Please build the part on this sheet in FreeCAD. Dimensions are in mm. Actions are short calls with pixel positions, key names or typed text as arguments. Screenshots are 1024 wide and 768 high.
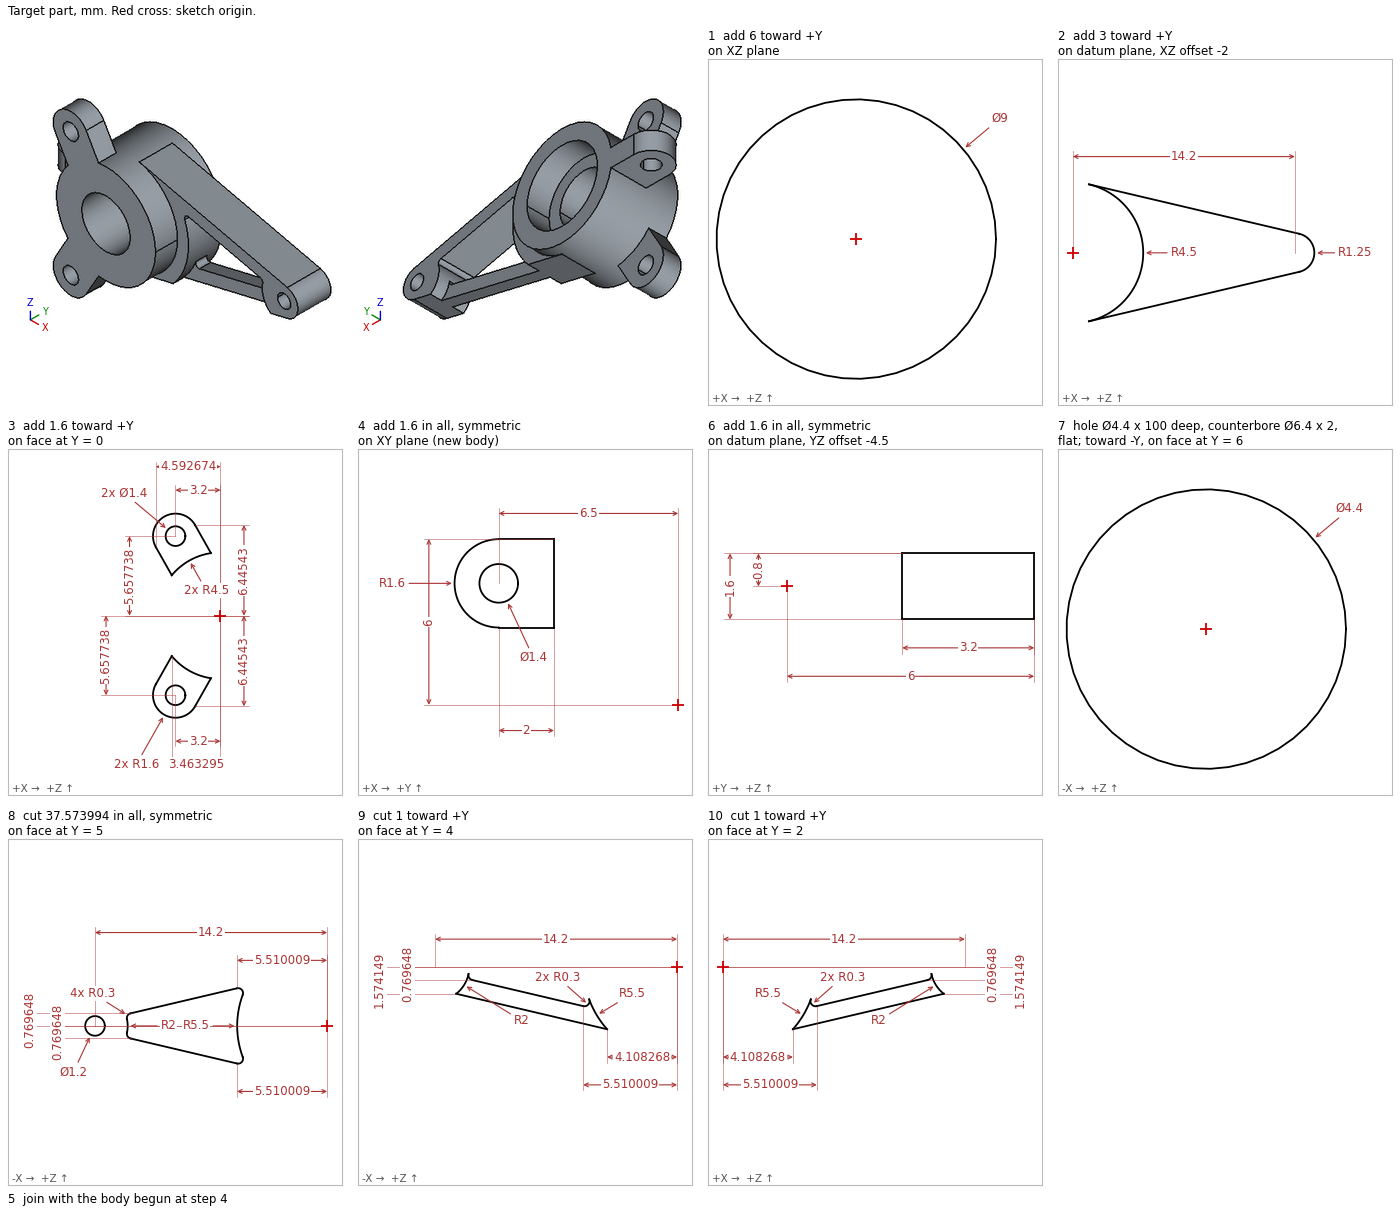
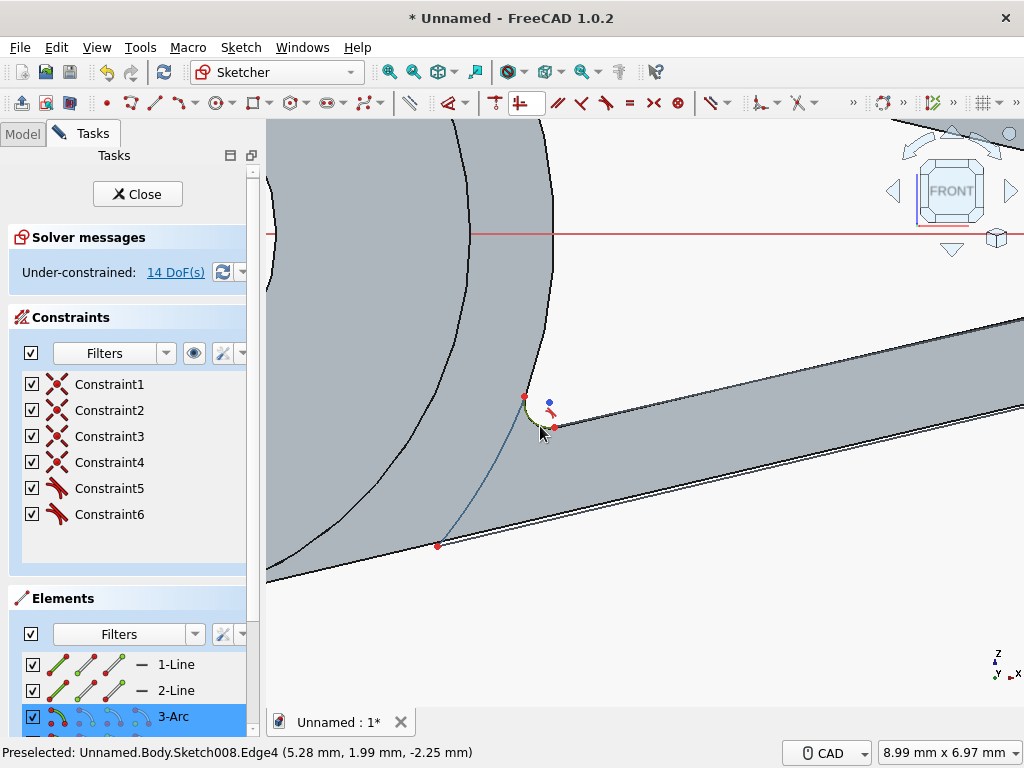
click(606, 104)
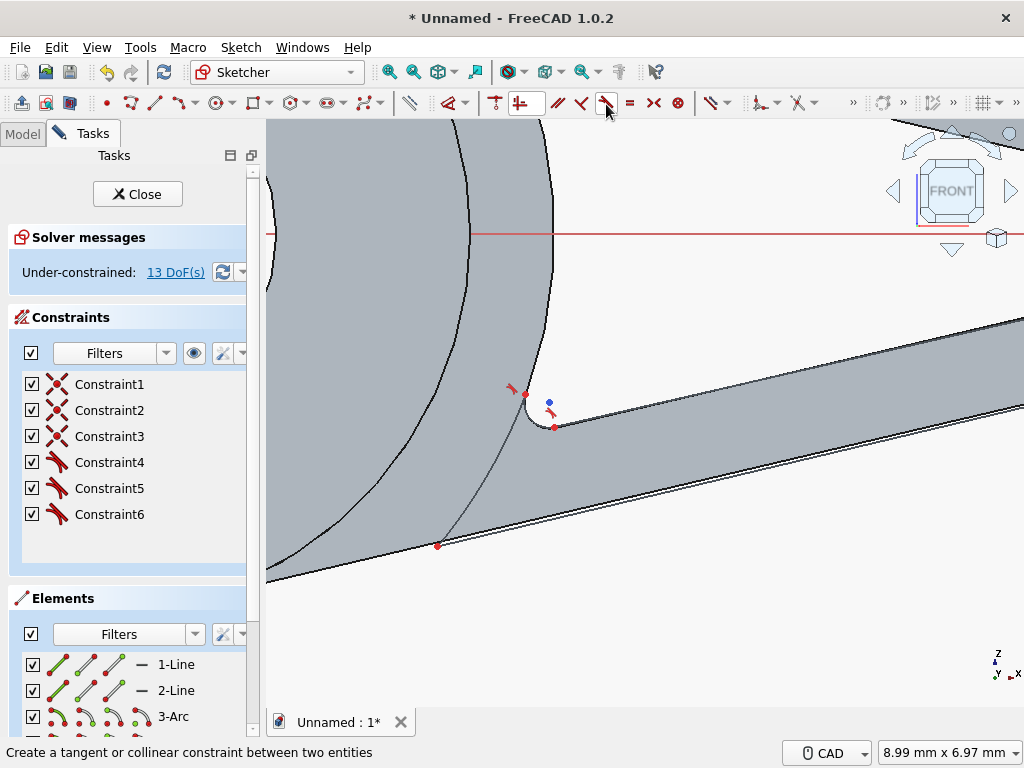
scroll(541, 427, down, 5)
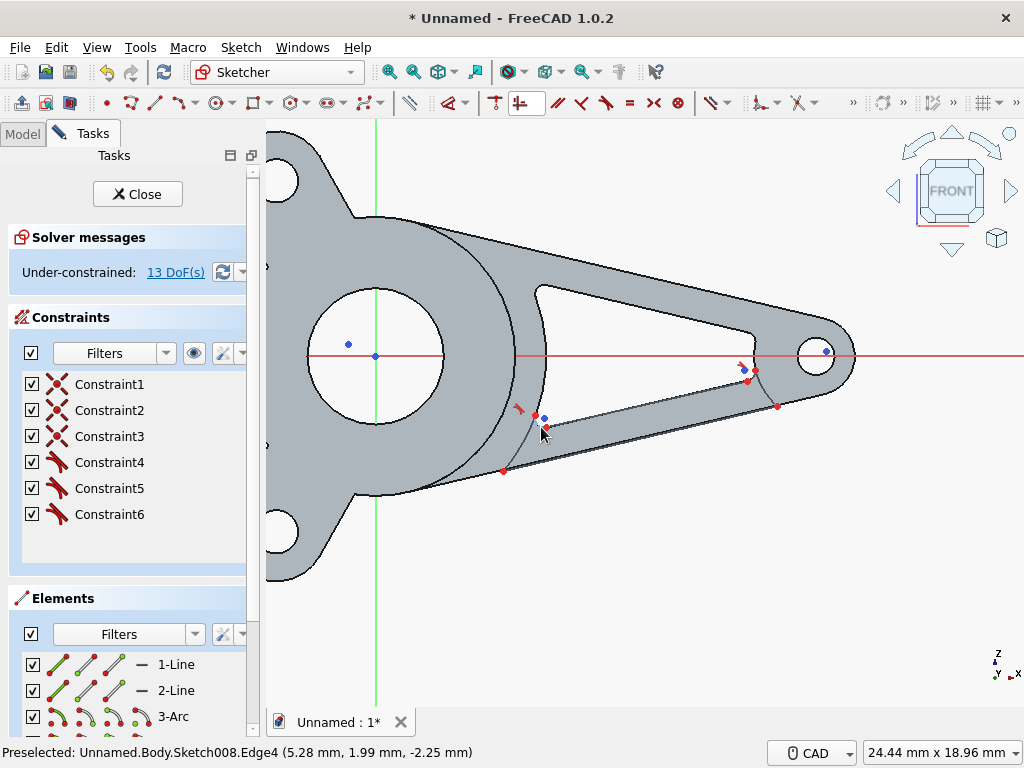
scroll(751, 379, up, 6)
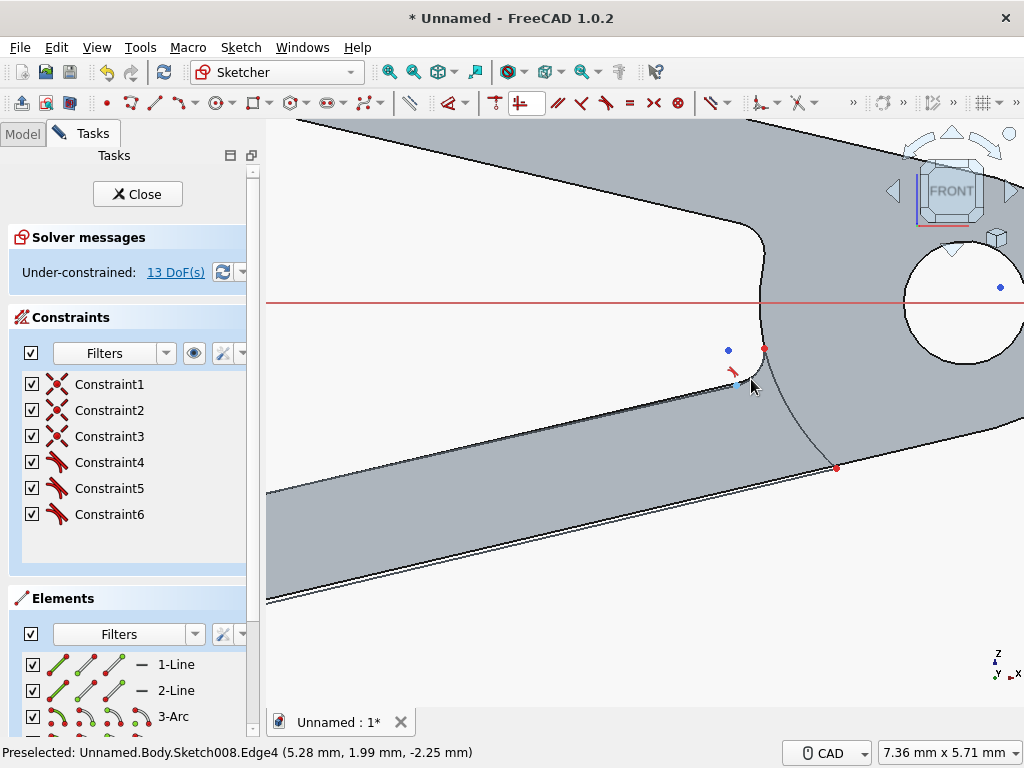
click(751, 379)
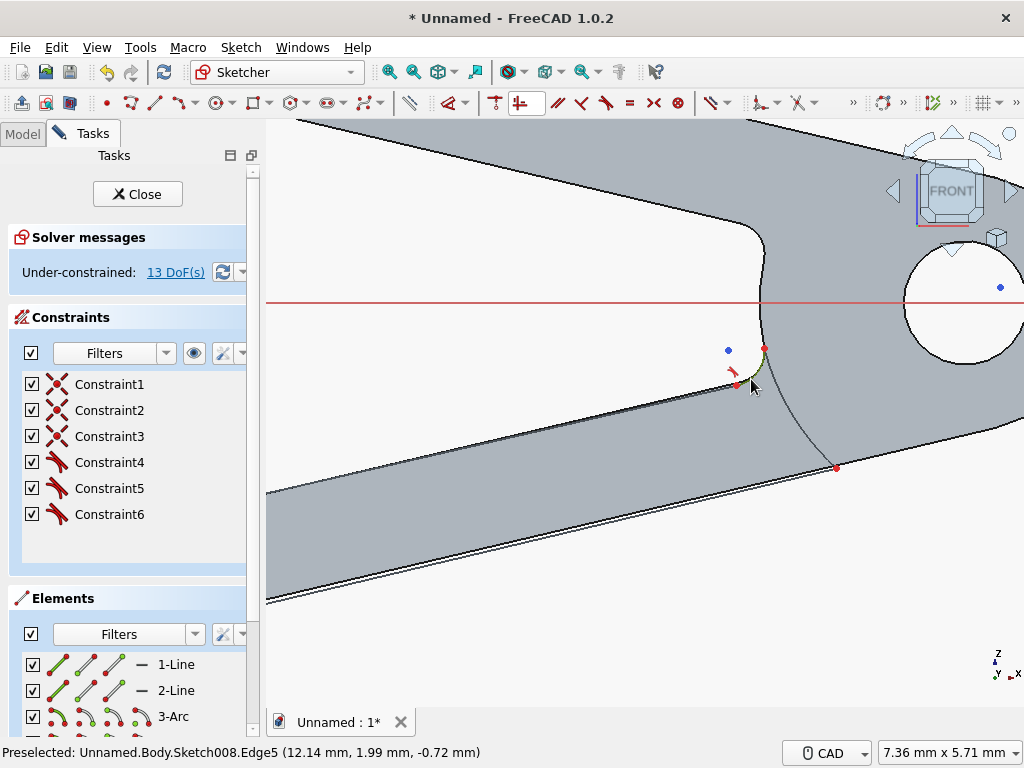
click(779, 389)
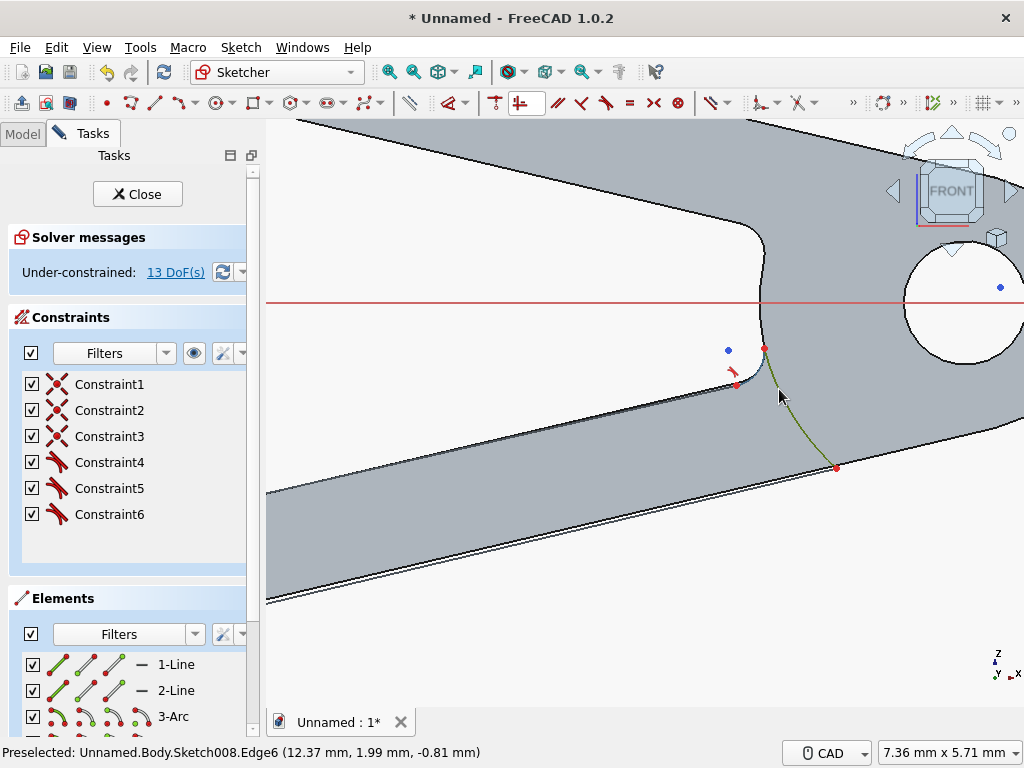
key(t)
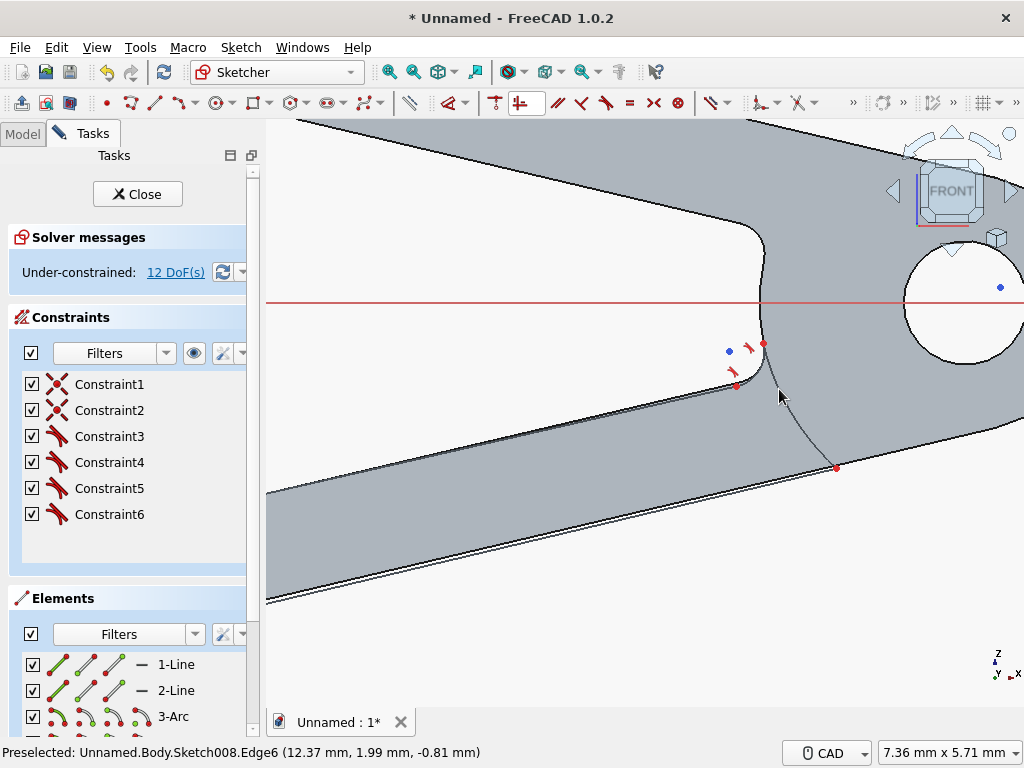
scroll(751, 379, down, 6)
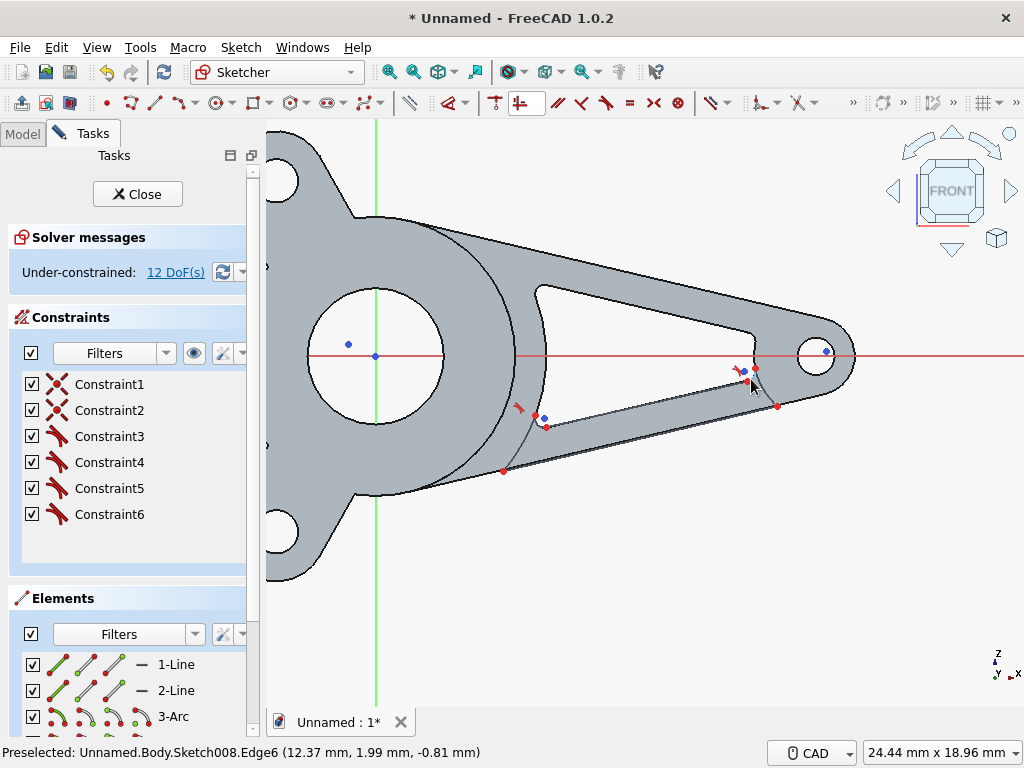
scroll(362, 350, up, 8)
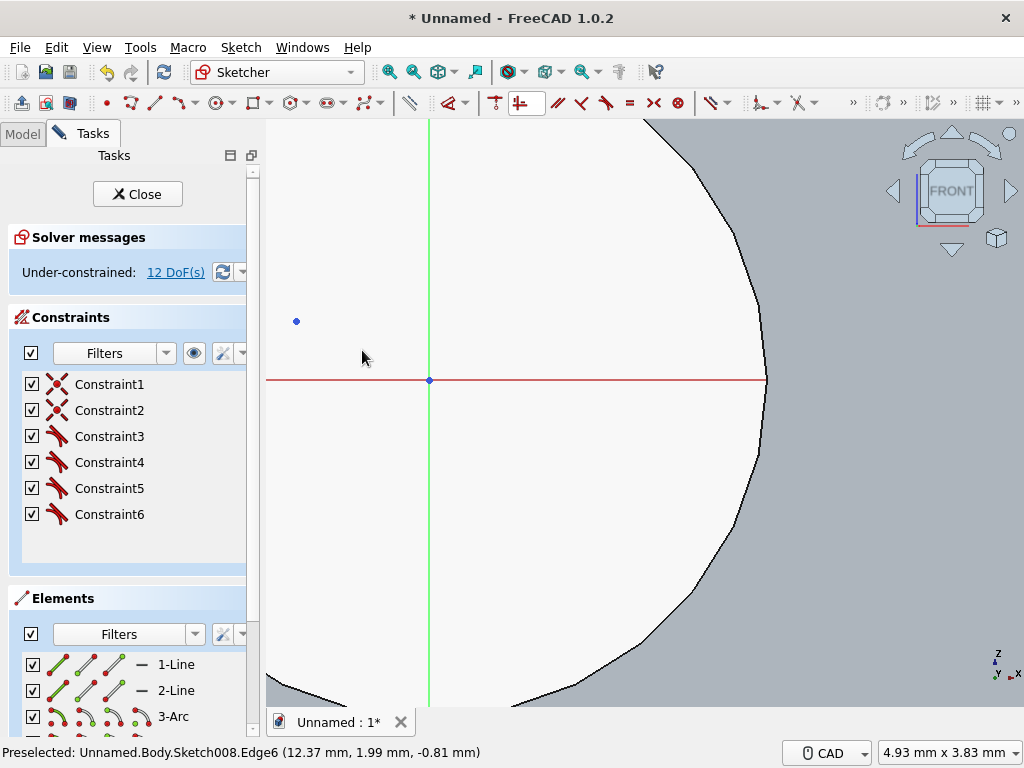
drag(286, 312, 439, 390)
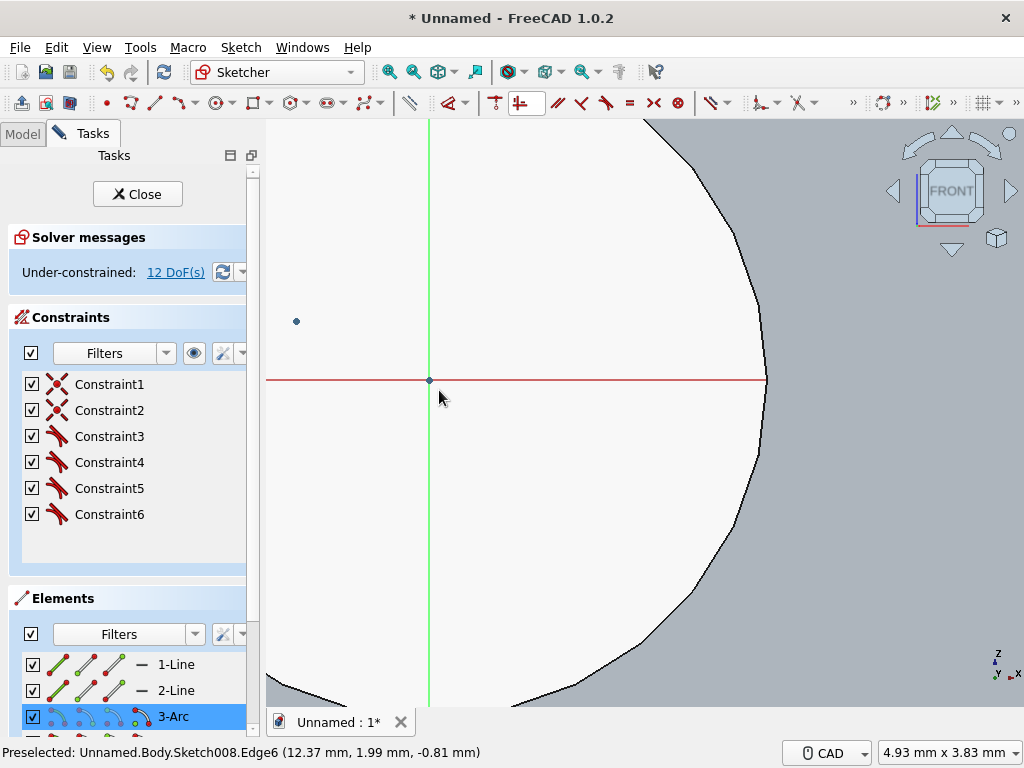
key(c)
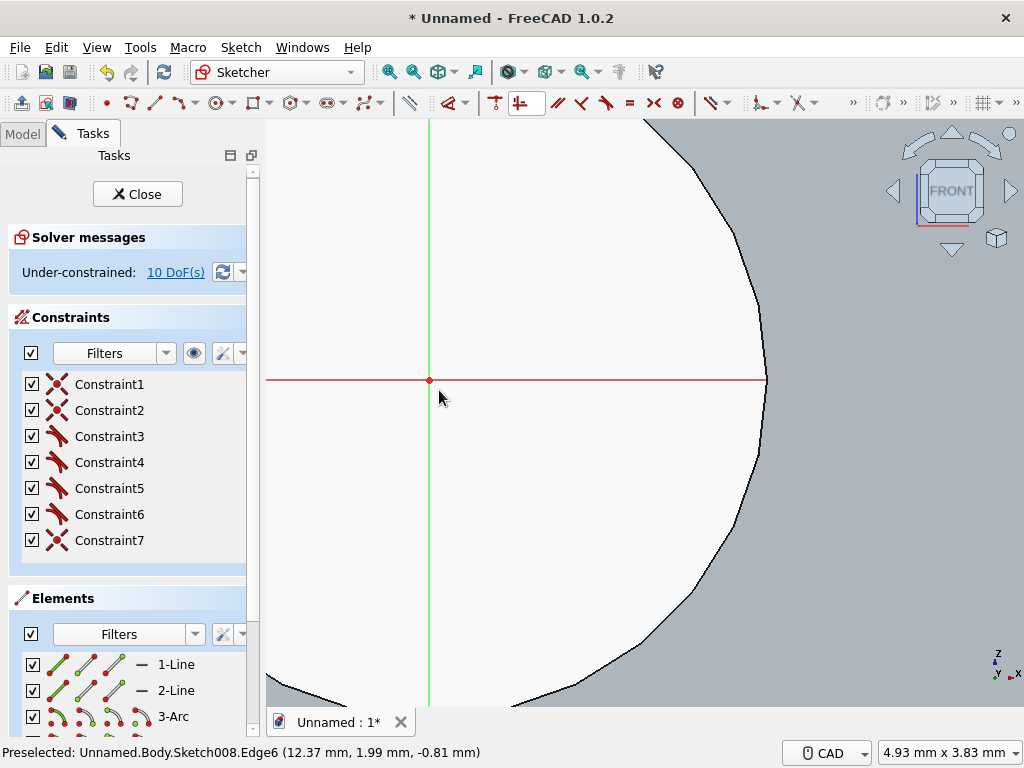
scroll(362, 350, down, 8)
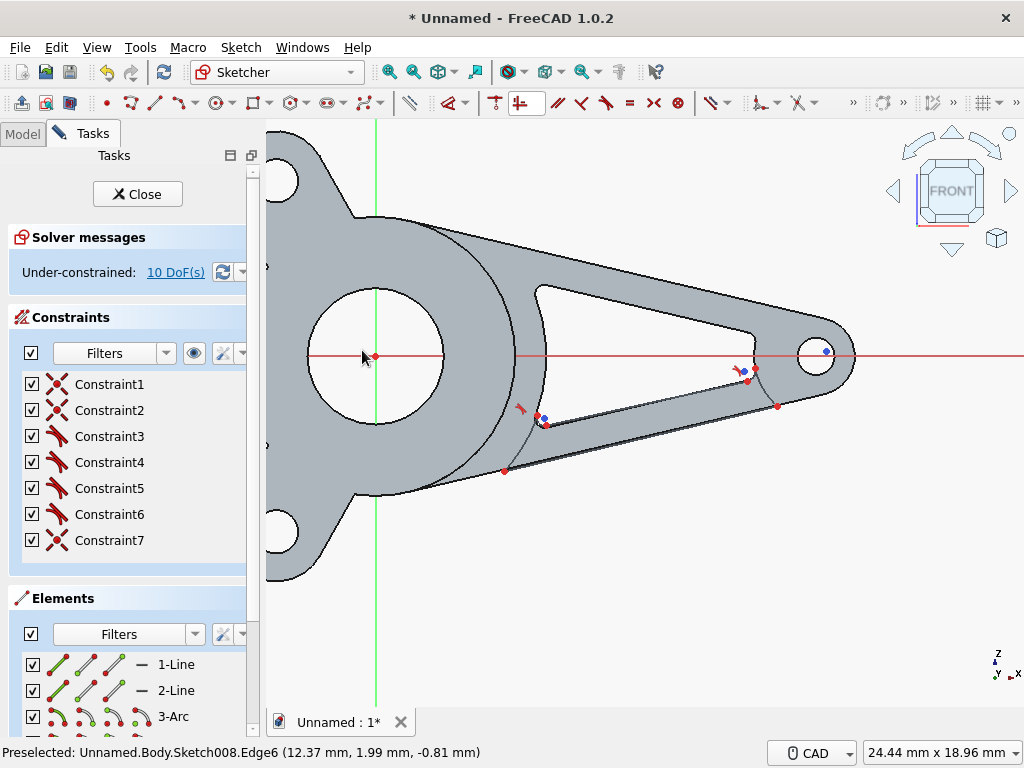
scroll(542, 425, up, 6)